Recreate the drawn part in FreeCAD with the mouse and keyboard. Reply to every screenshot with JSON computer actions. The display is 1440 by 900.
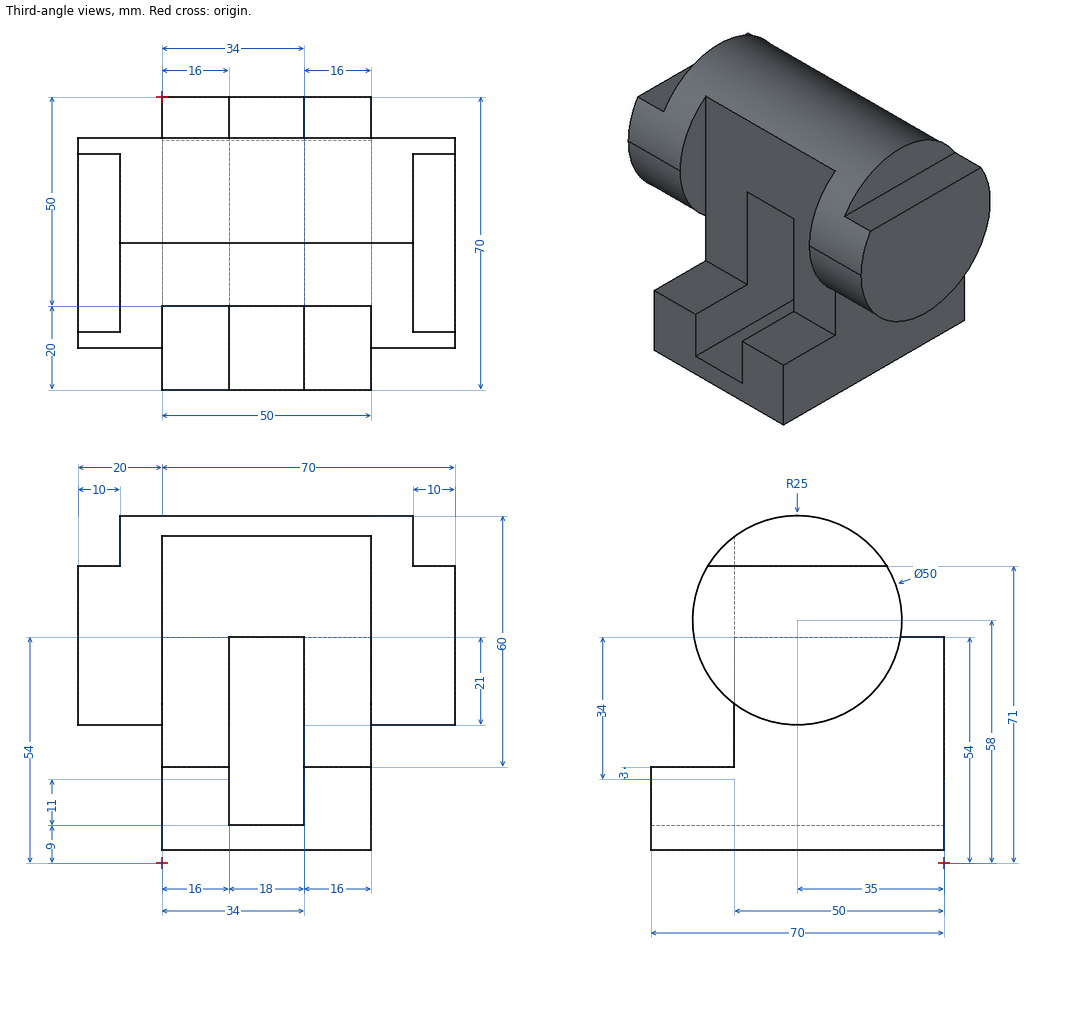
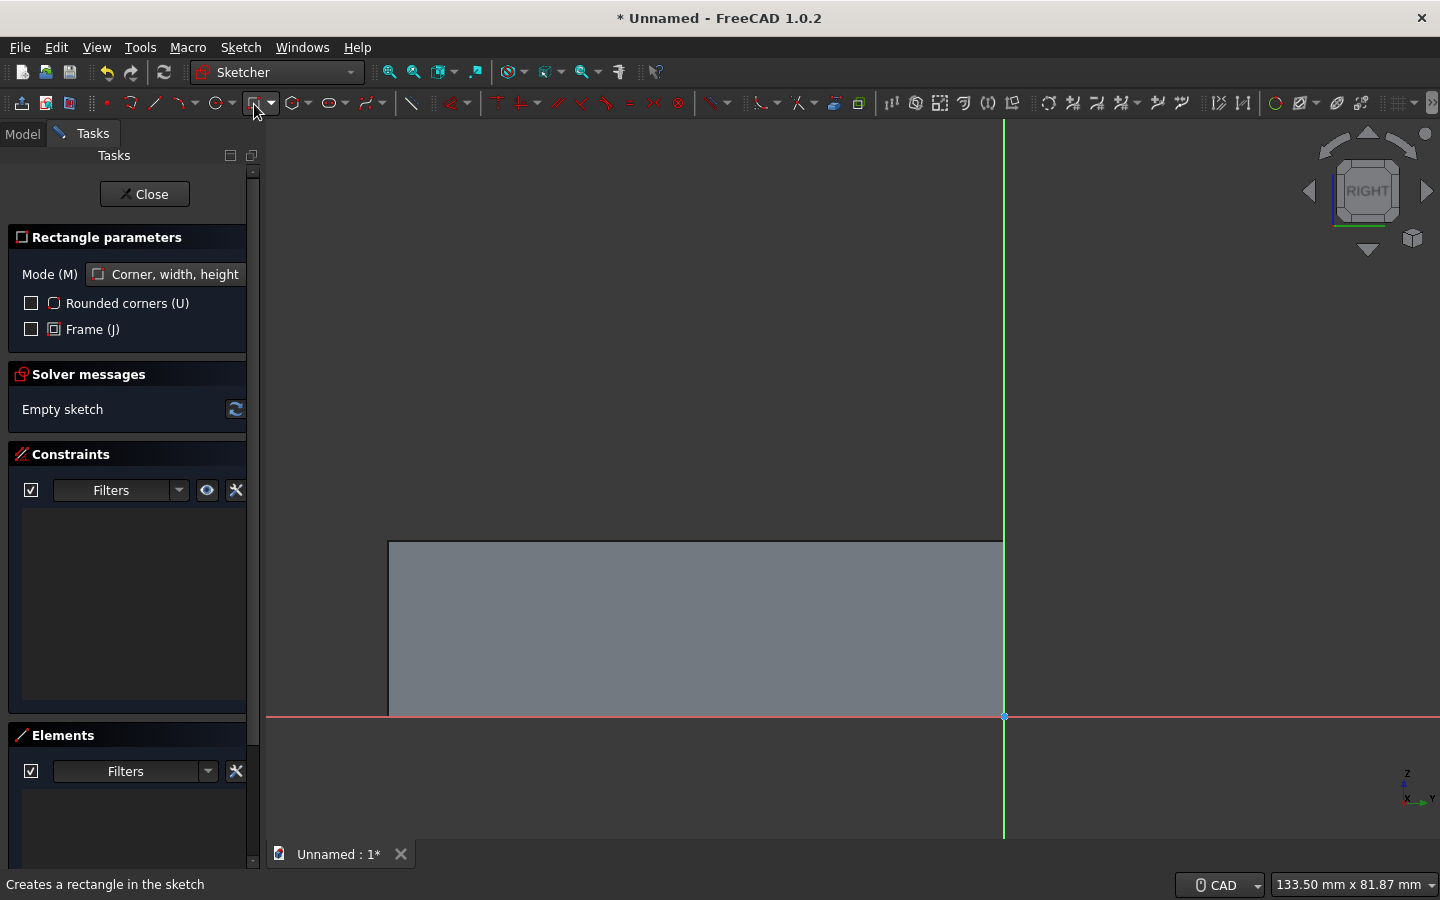
{"action": "left_click", "coordinate": [564, 242]}
{"action": "left_click", "coordinate": [1004, 541]}
{"action": "key", "text": "Escape"}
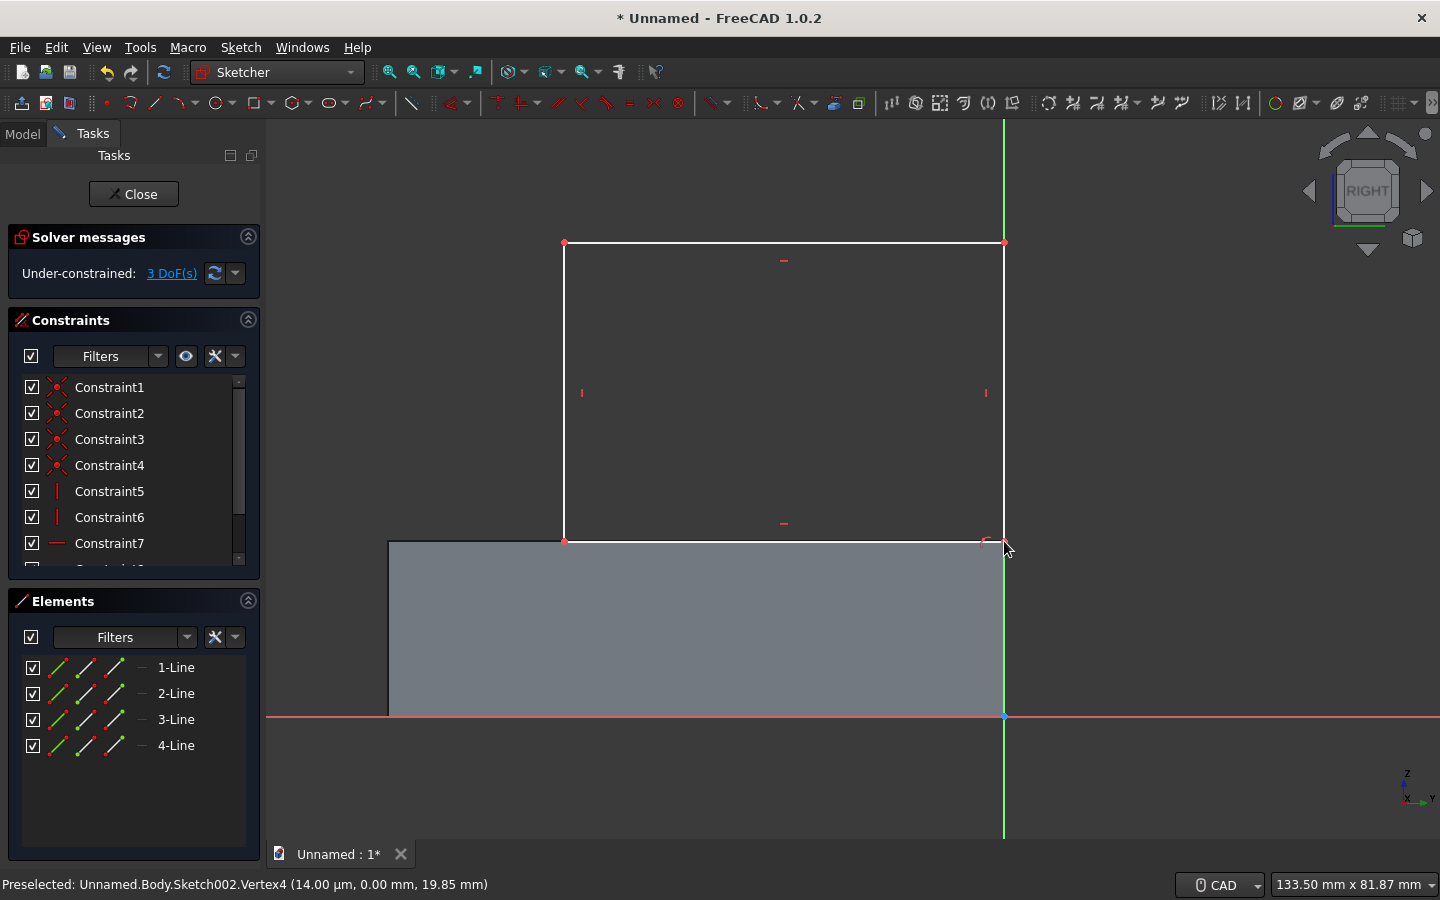
{"action": "left_click", "coordinate": [564, 333]}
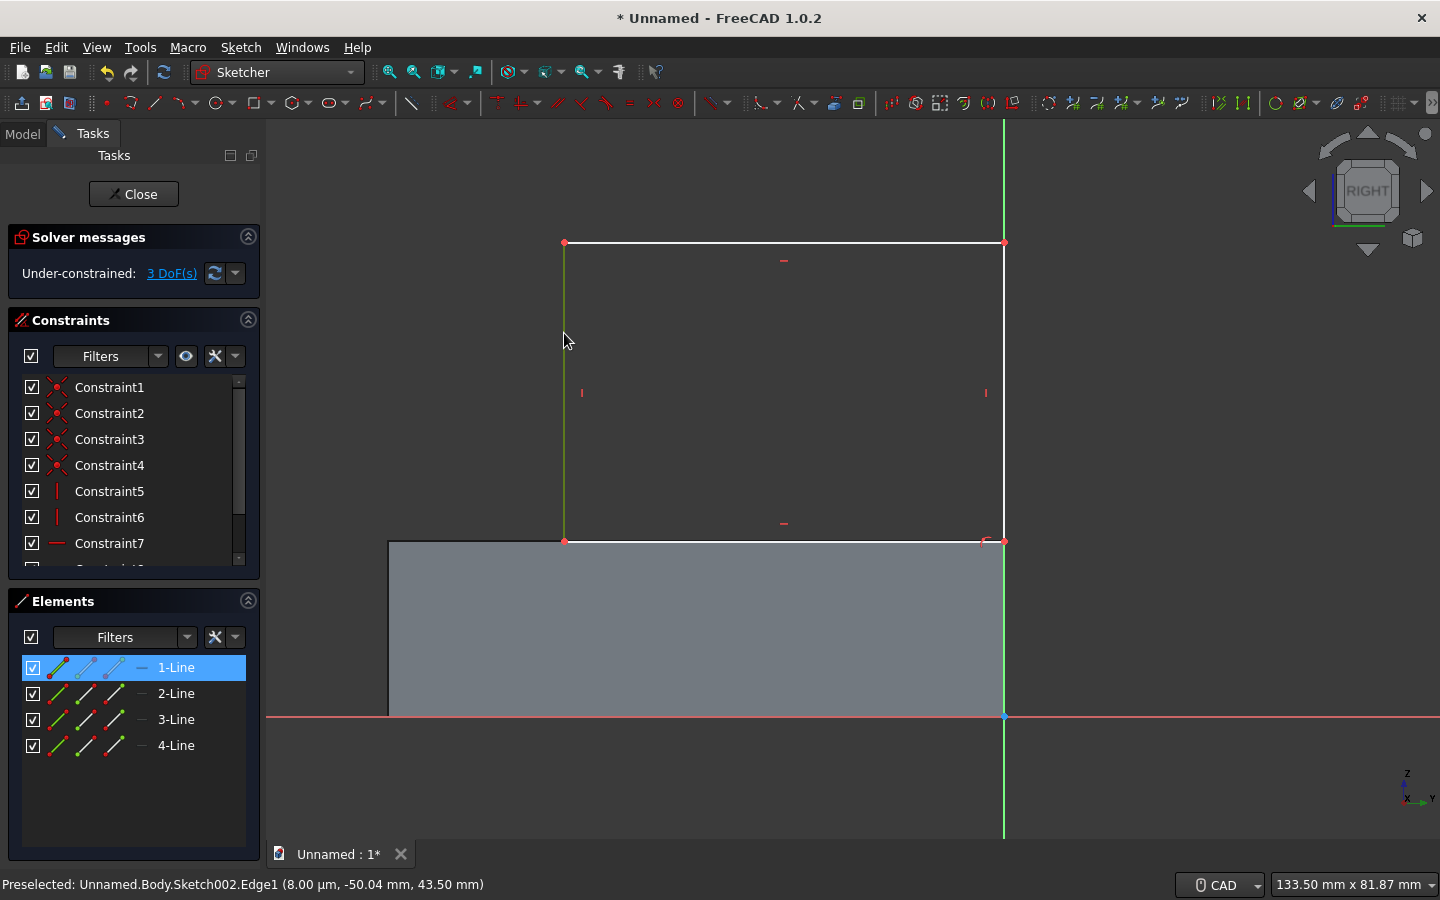
{"action": "key", "text": "i"}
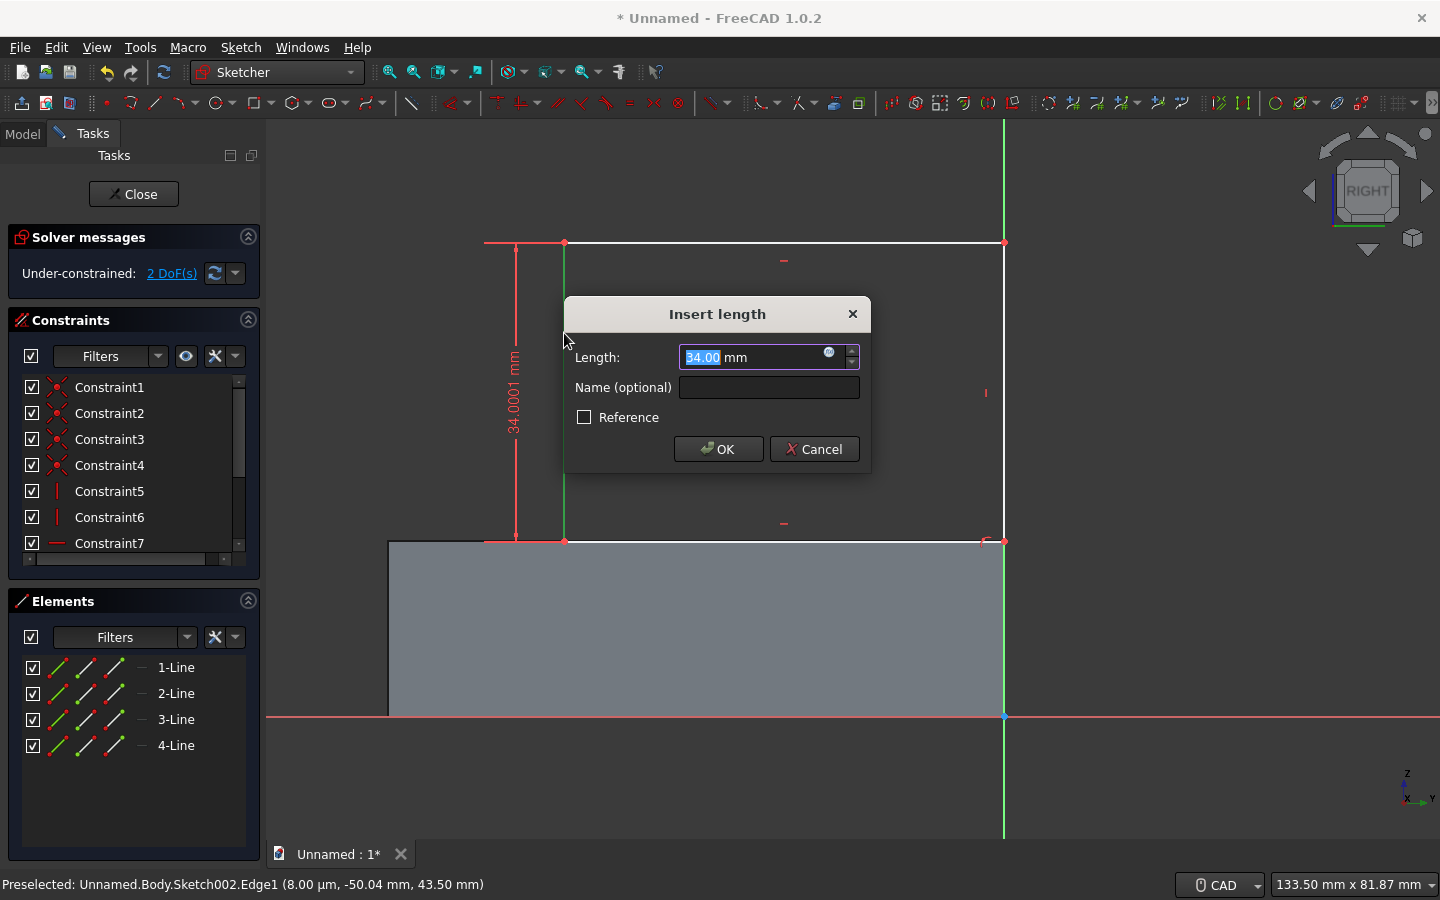
{"action": "type", "text": "34"}
{"action": "key", "text": "Return"}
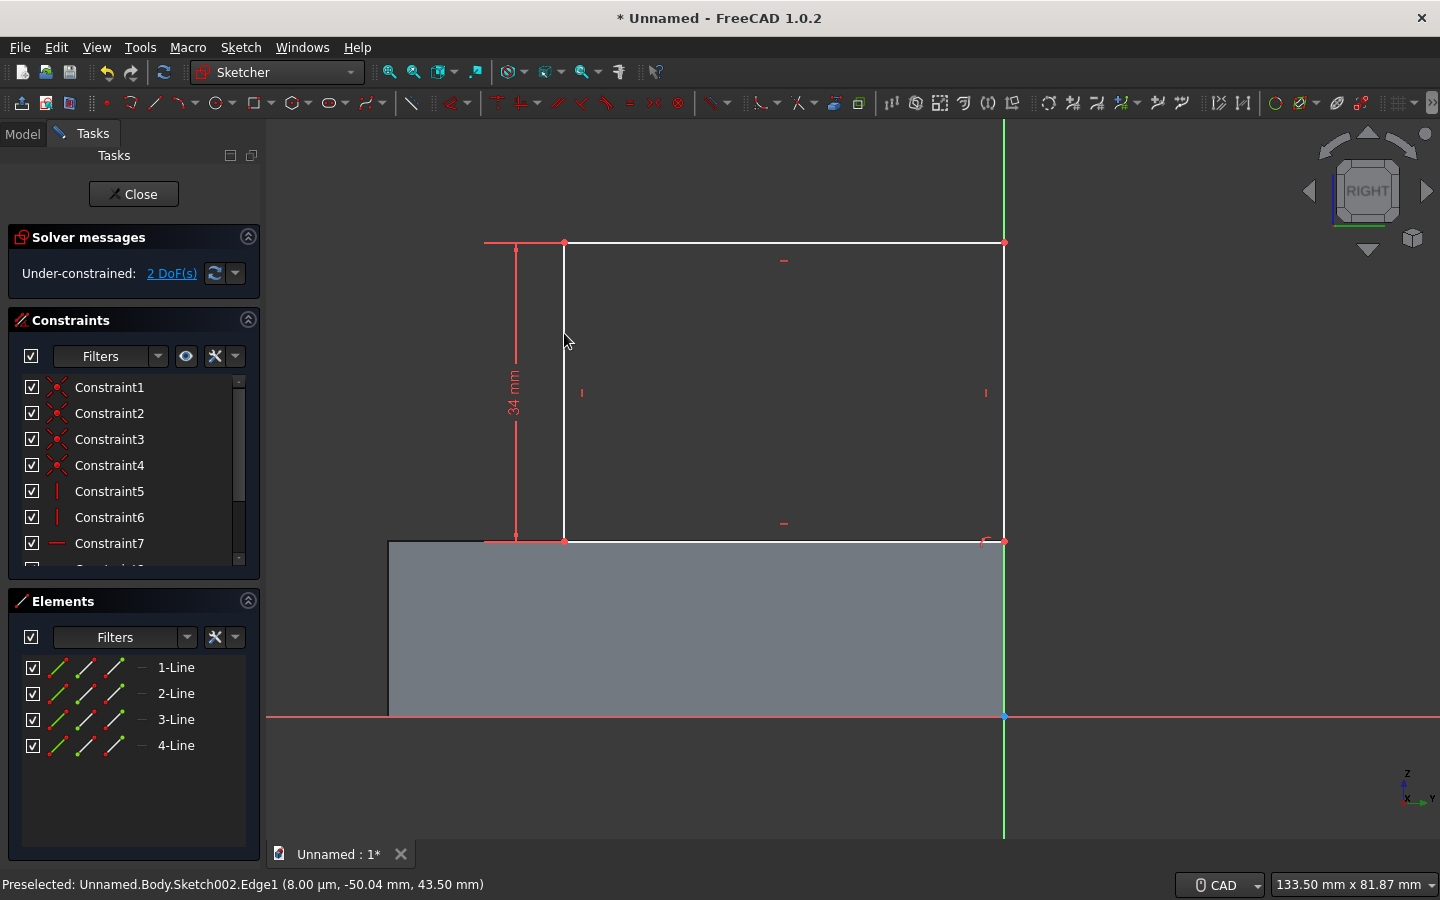
{"action": "left_click", "coordinate": [696, 542]}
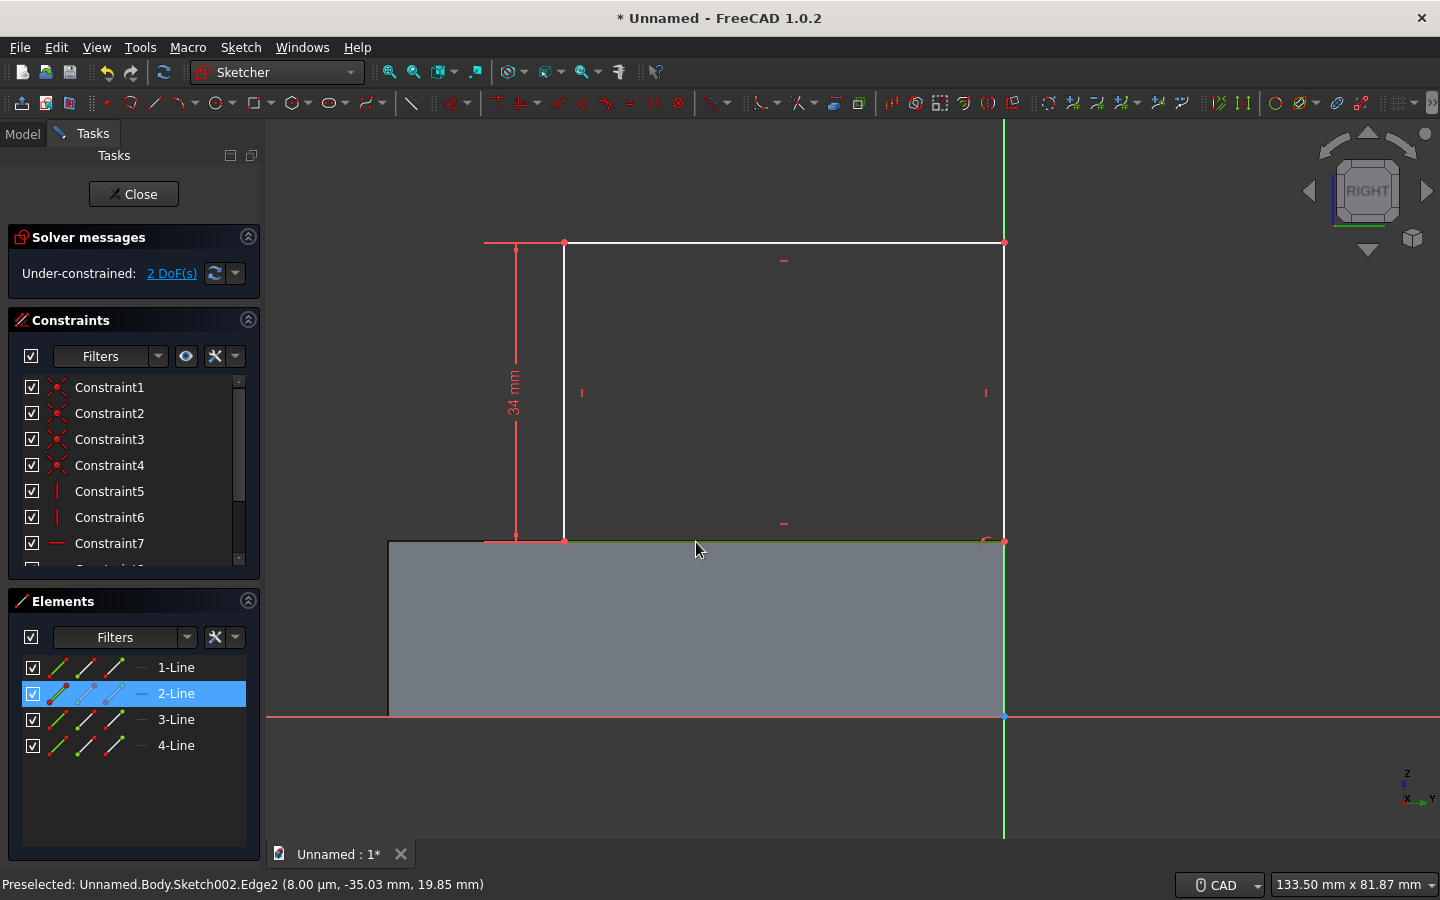
{"action": "key", "text": "l"}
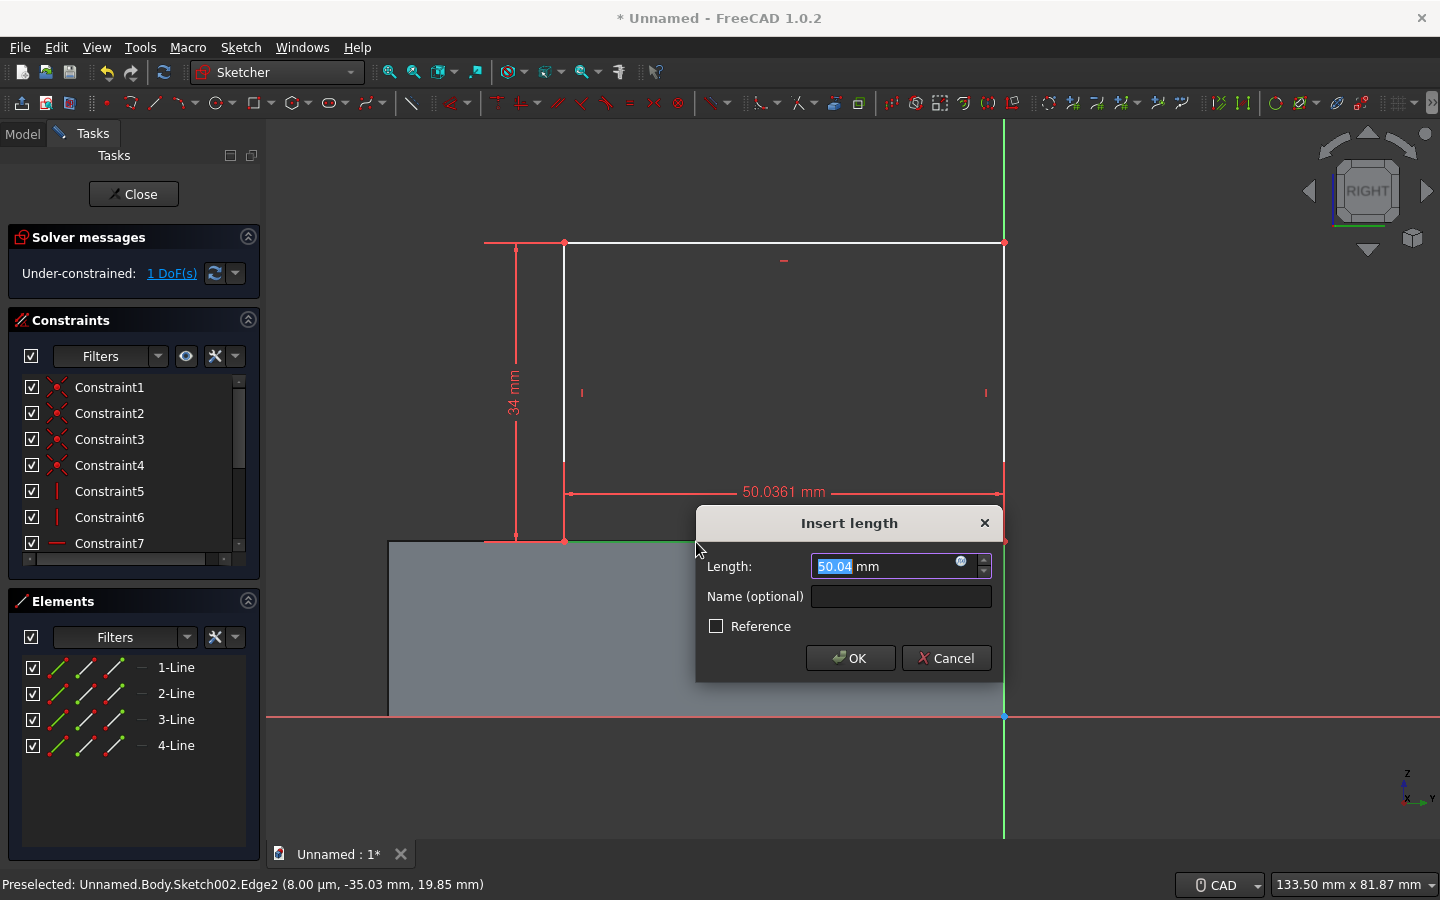
{"action": "type", "text": "50"}
{"action": "key", "text": "Return"}